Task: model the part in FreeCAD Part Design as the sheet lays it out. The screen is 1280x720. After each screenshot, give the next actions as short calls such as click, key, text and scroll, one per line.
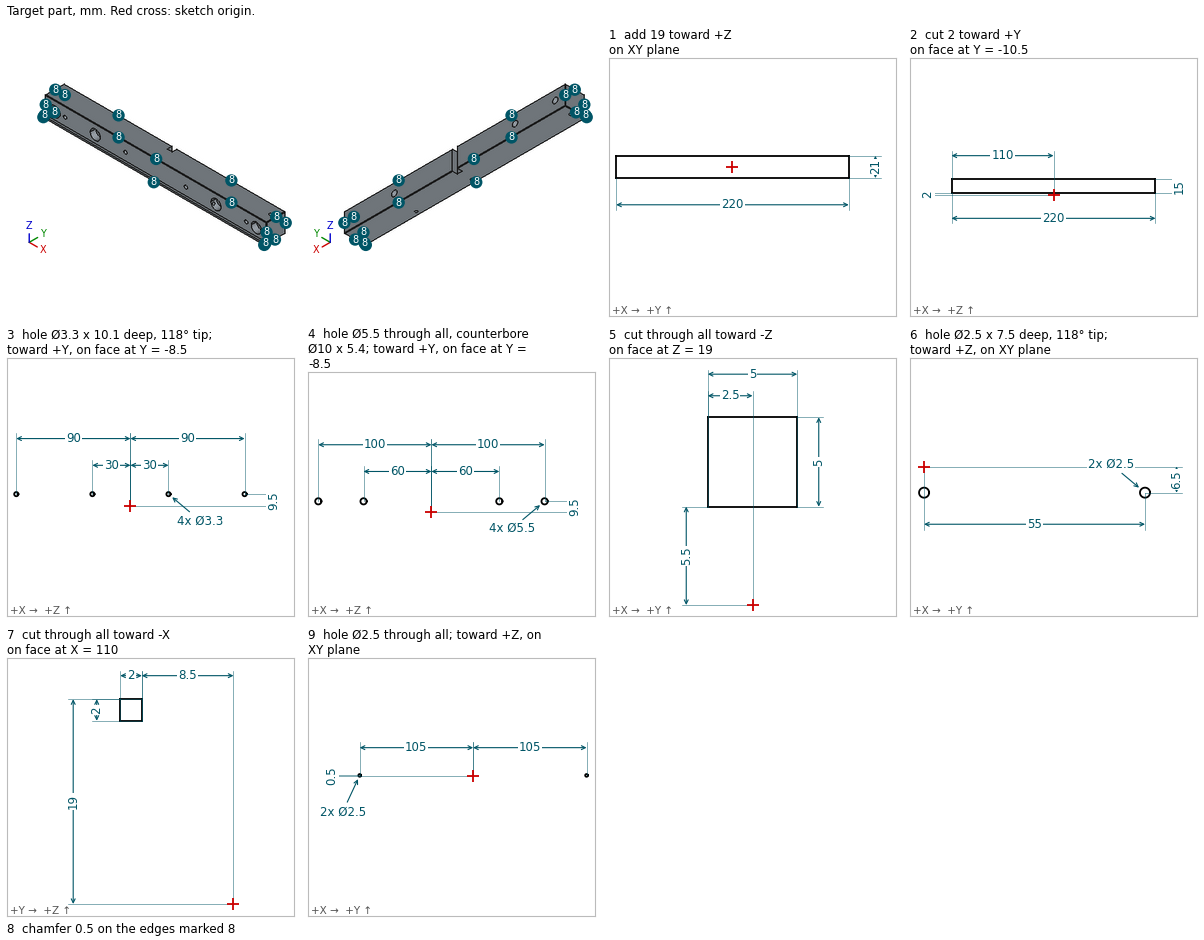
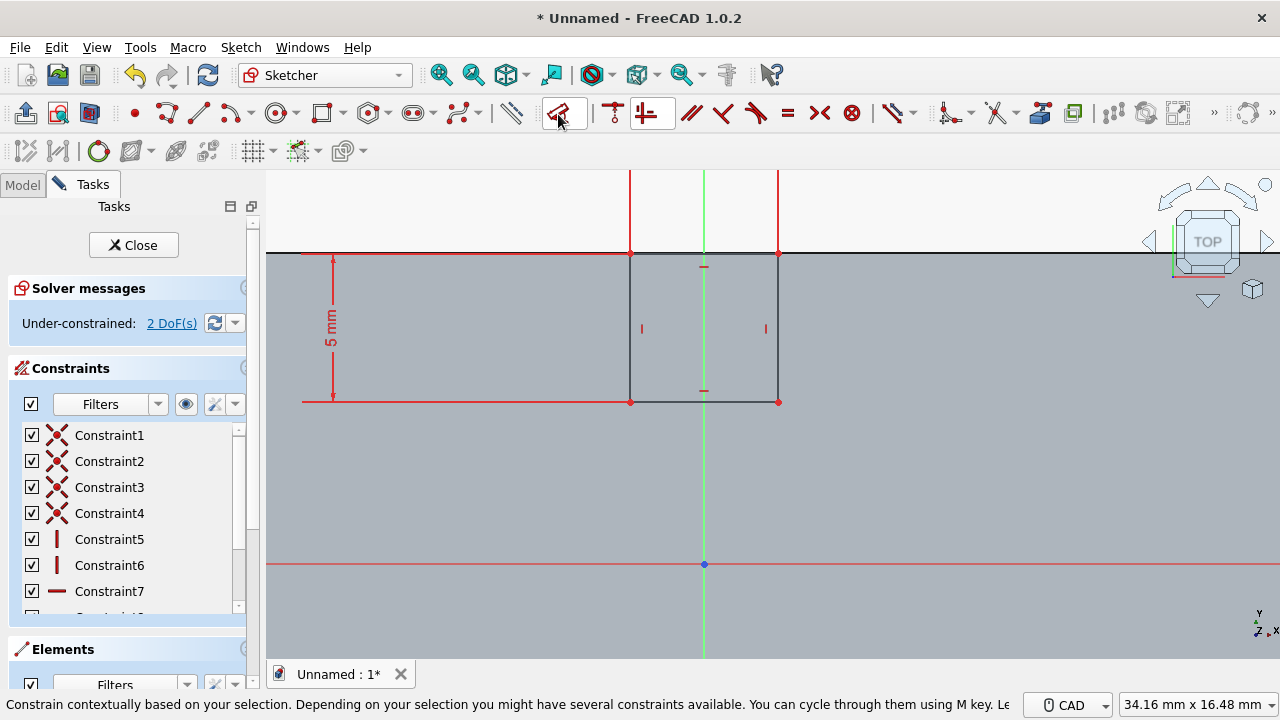
click(630, 254)
click(667, 598)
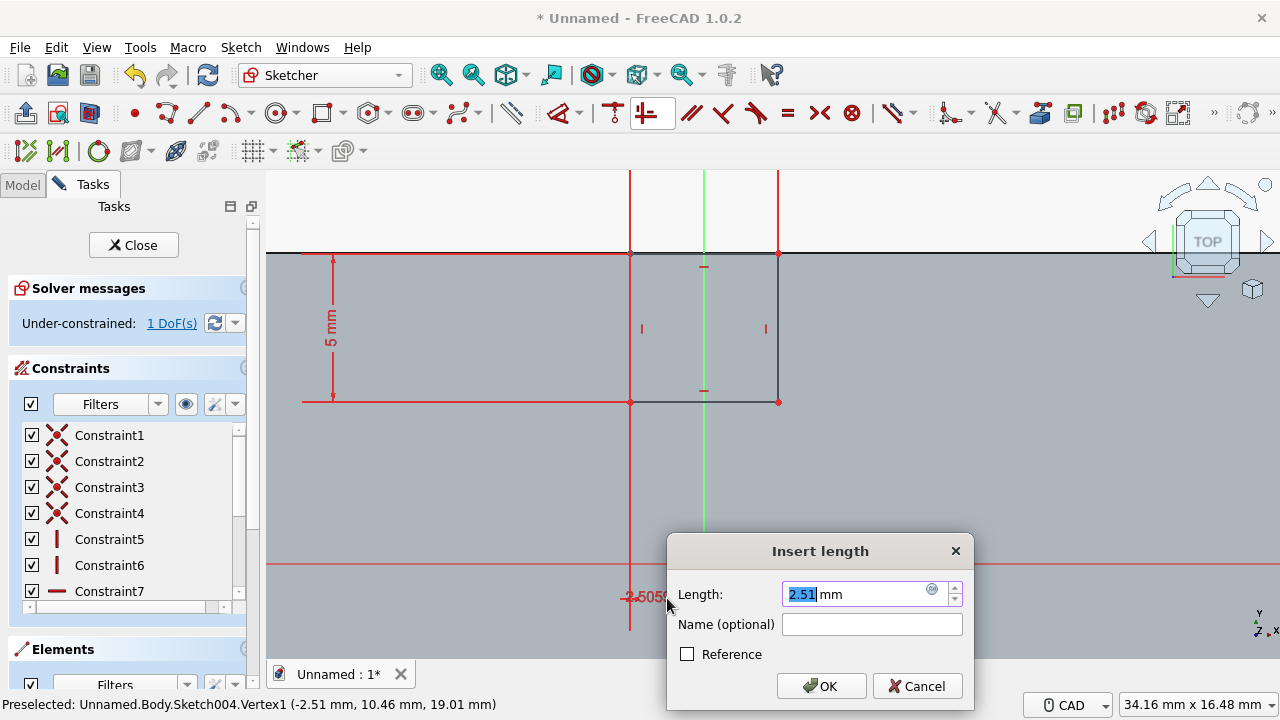
text(2.5)
key(Return)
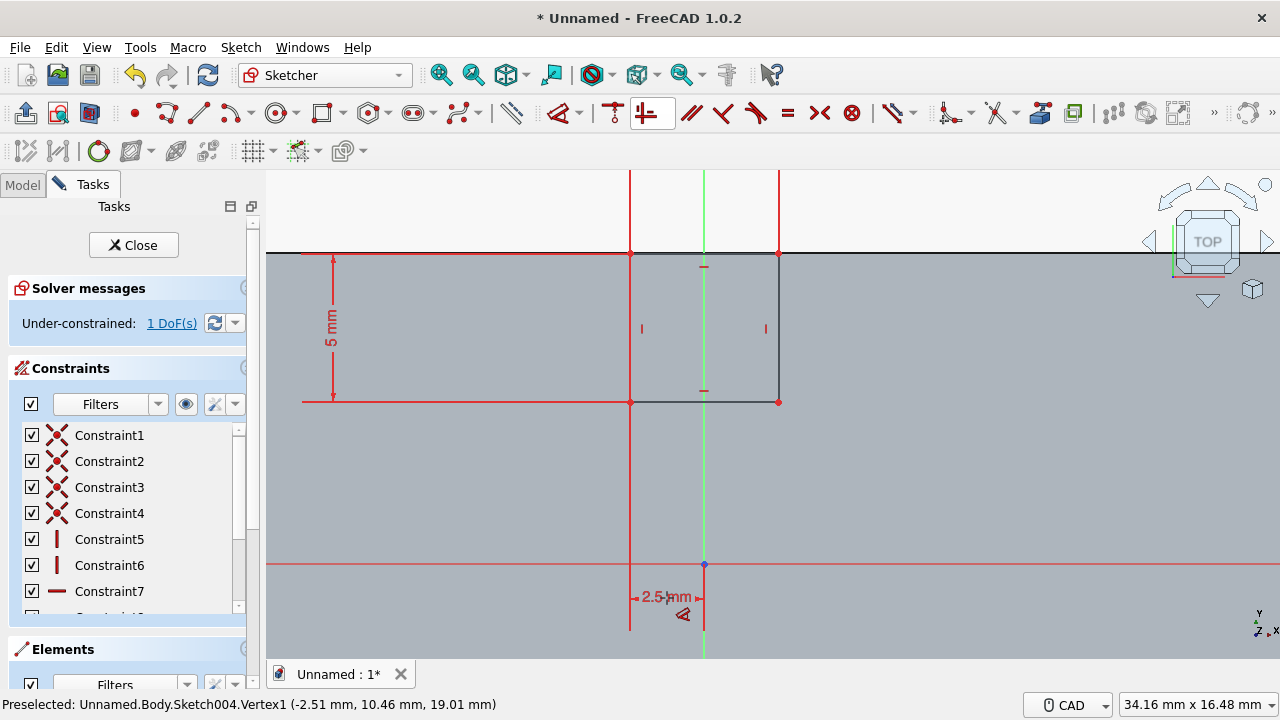
click(630, 402)
click(596, 483)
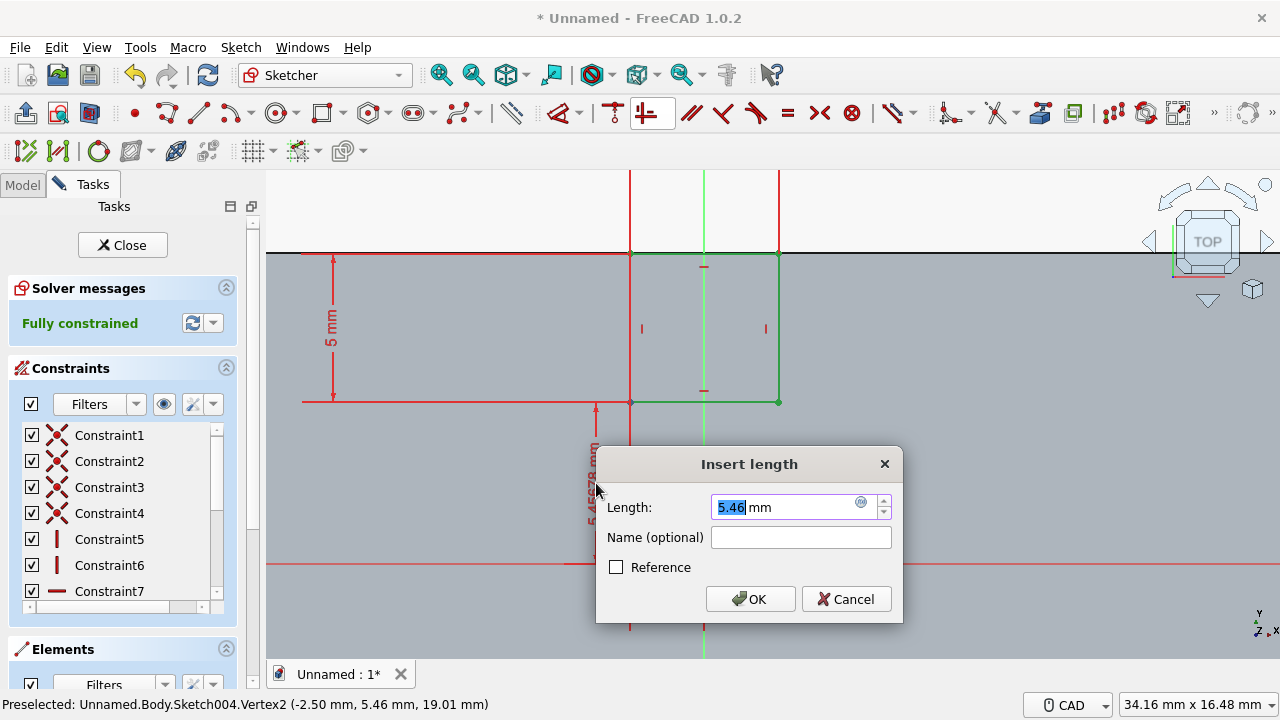
text(5.5)
key(Return)
key(Escape)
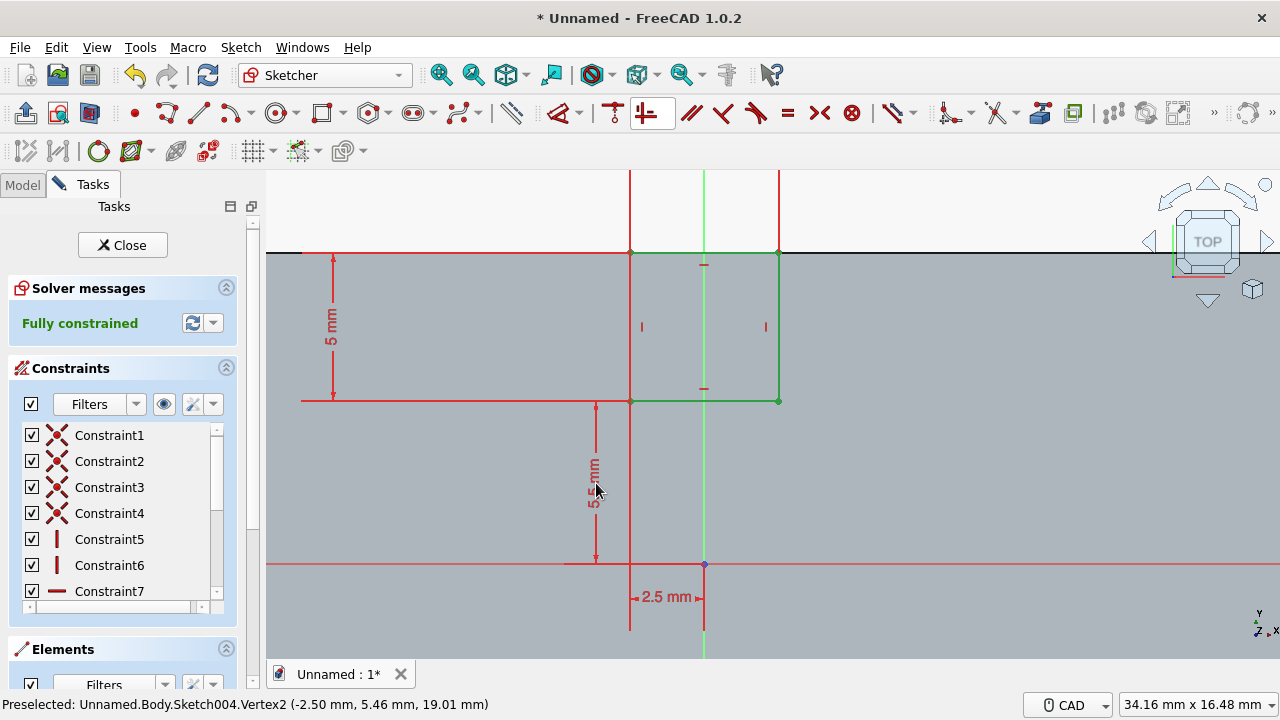
click(123, 245)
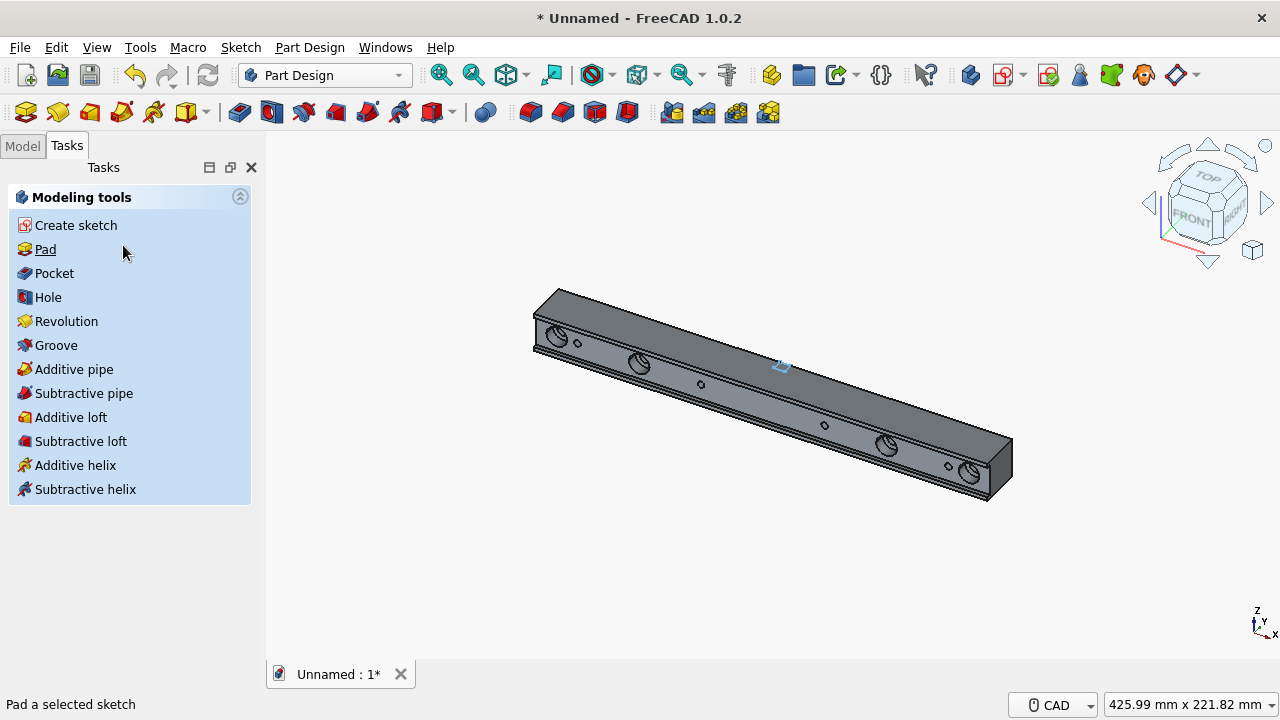
click(240, 112)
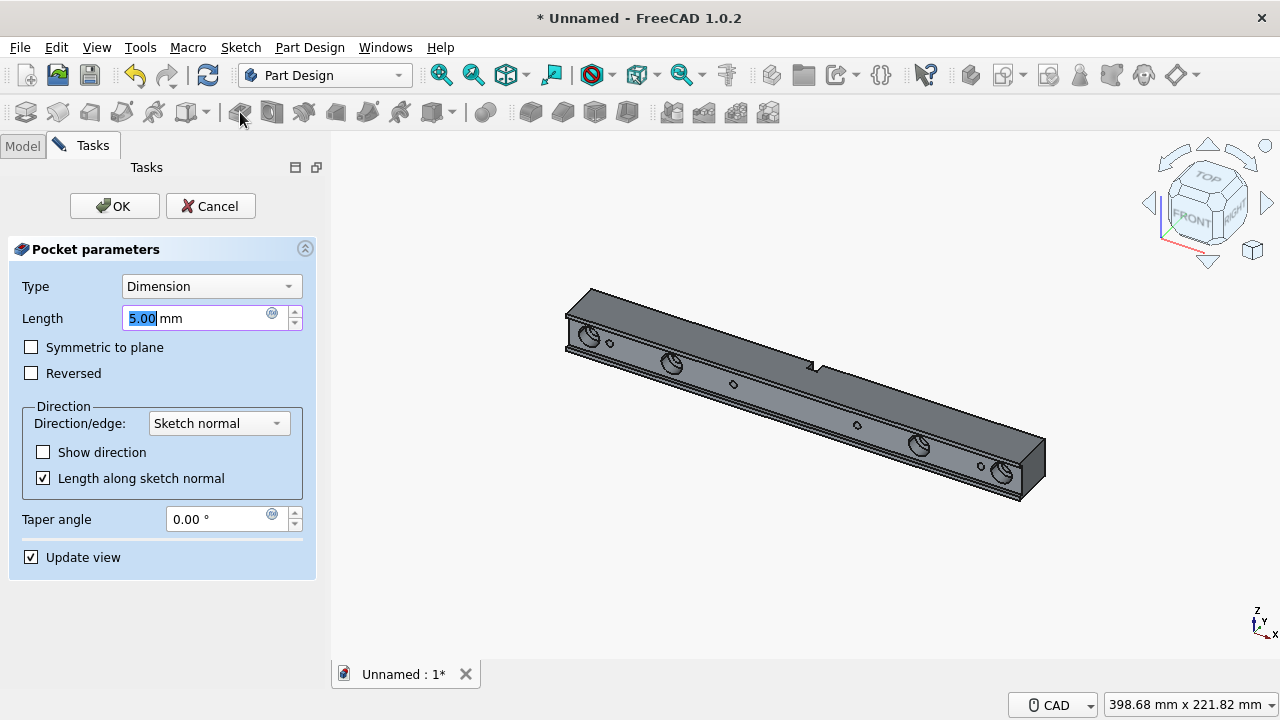
click(212, 286)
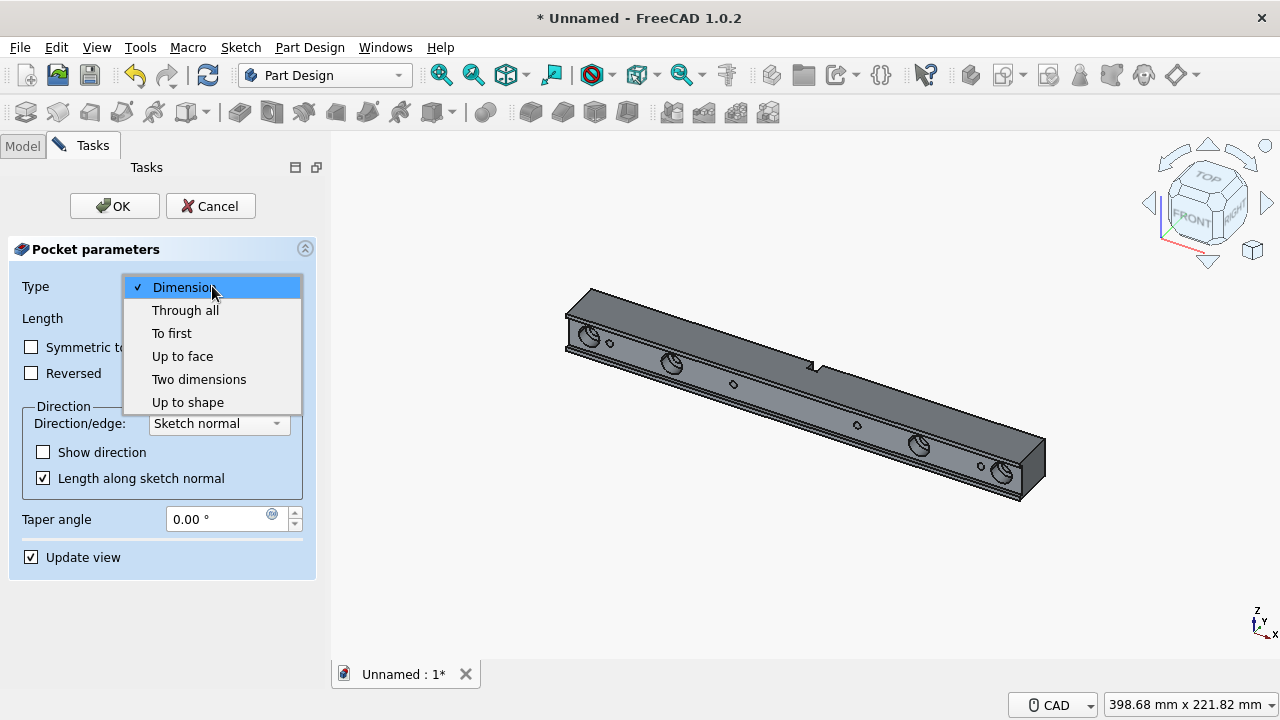
click(212, 310)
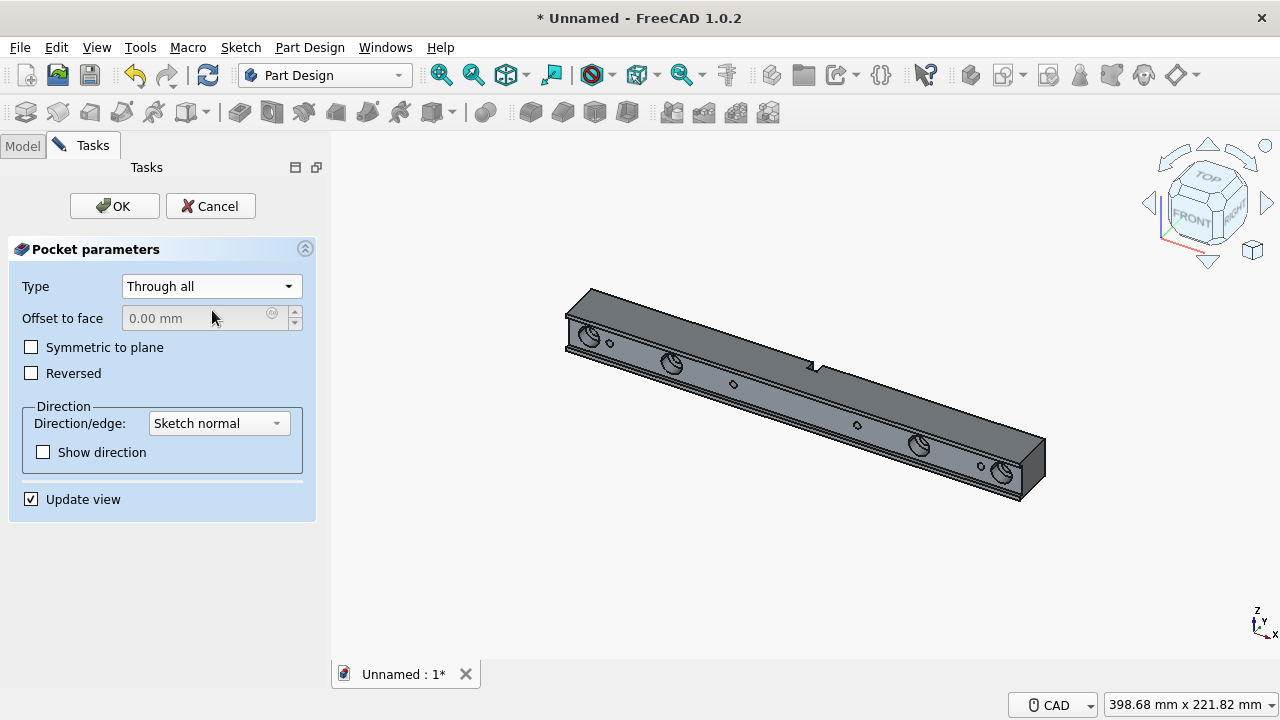
click(115, 206)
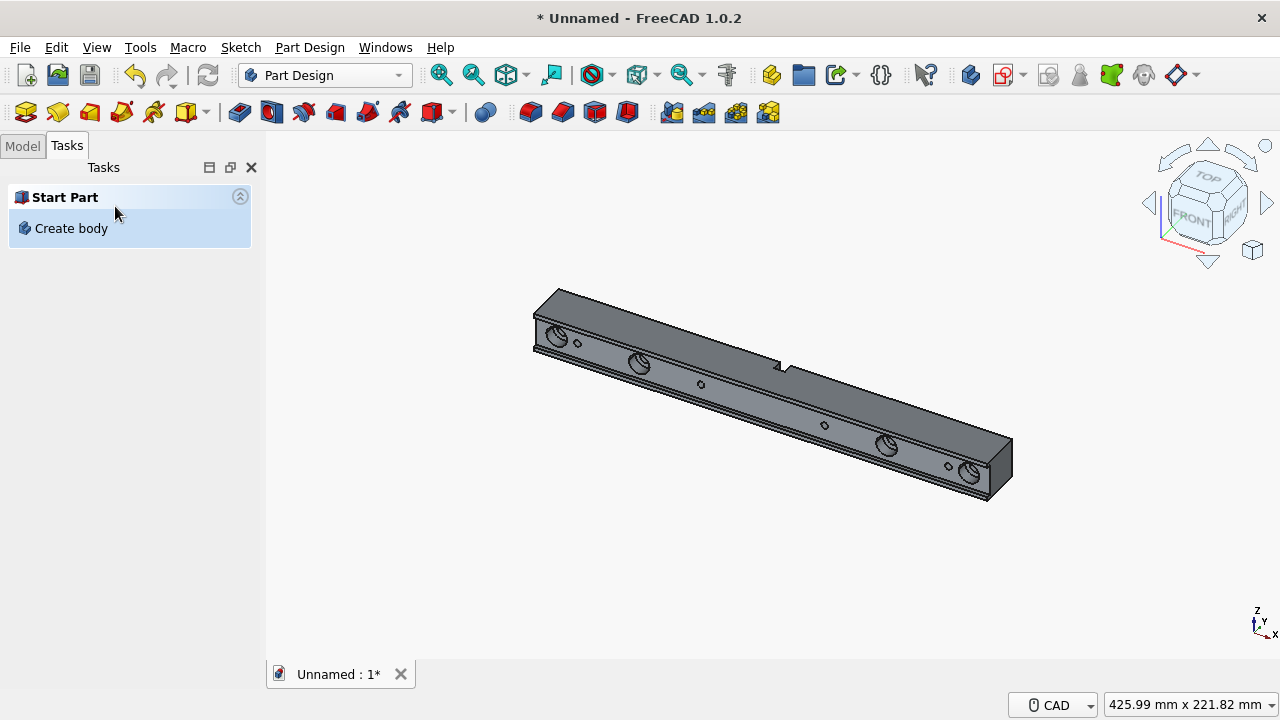
click(1004, 76)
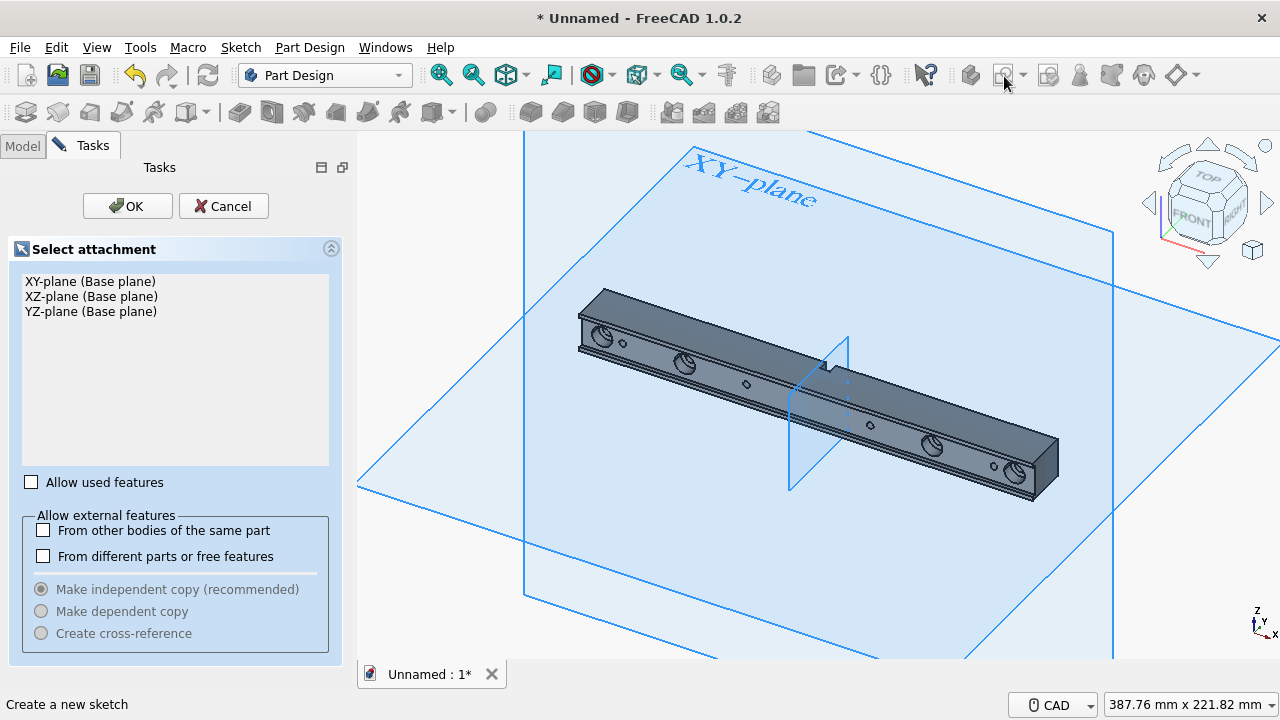
click(82, 282)